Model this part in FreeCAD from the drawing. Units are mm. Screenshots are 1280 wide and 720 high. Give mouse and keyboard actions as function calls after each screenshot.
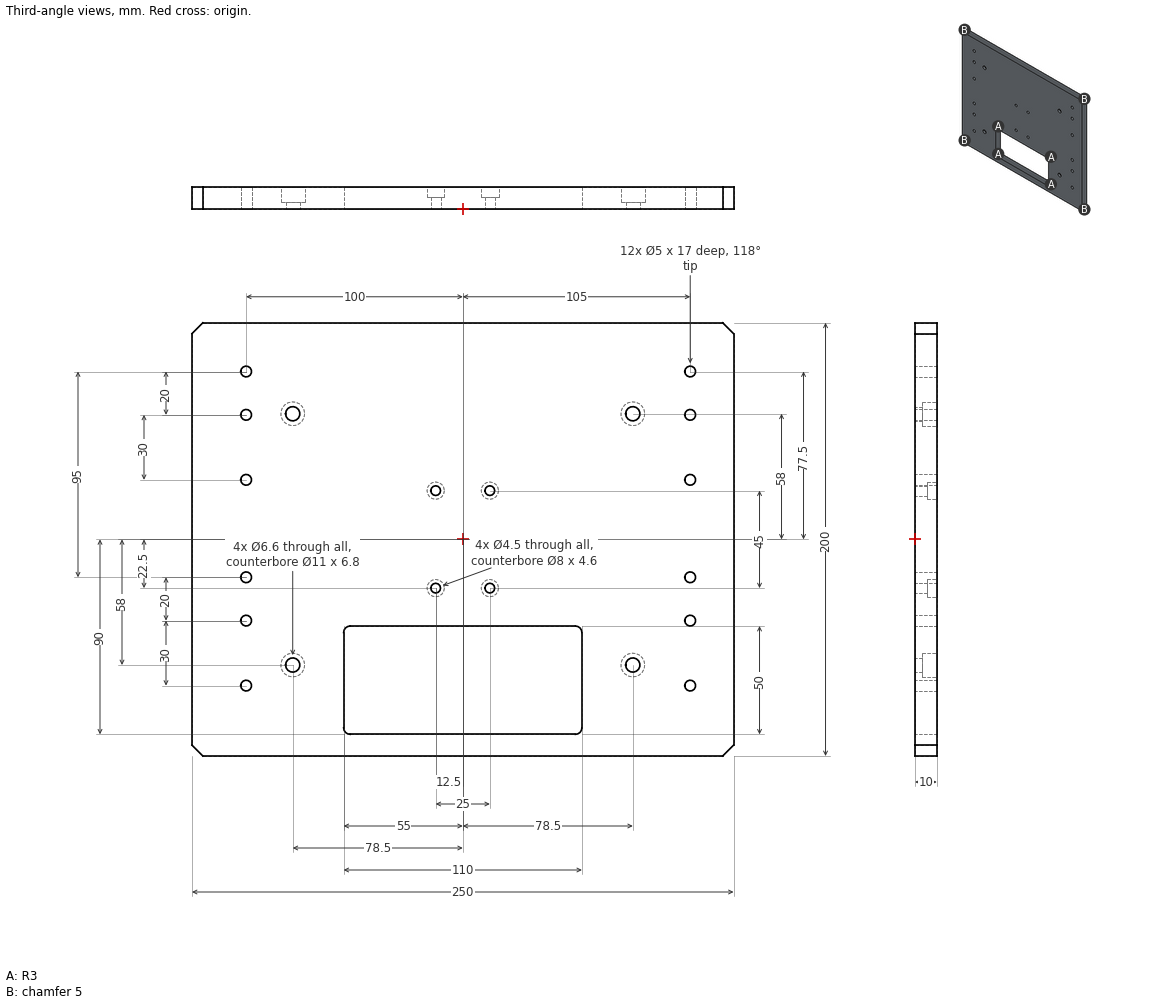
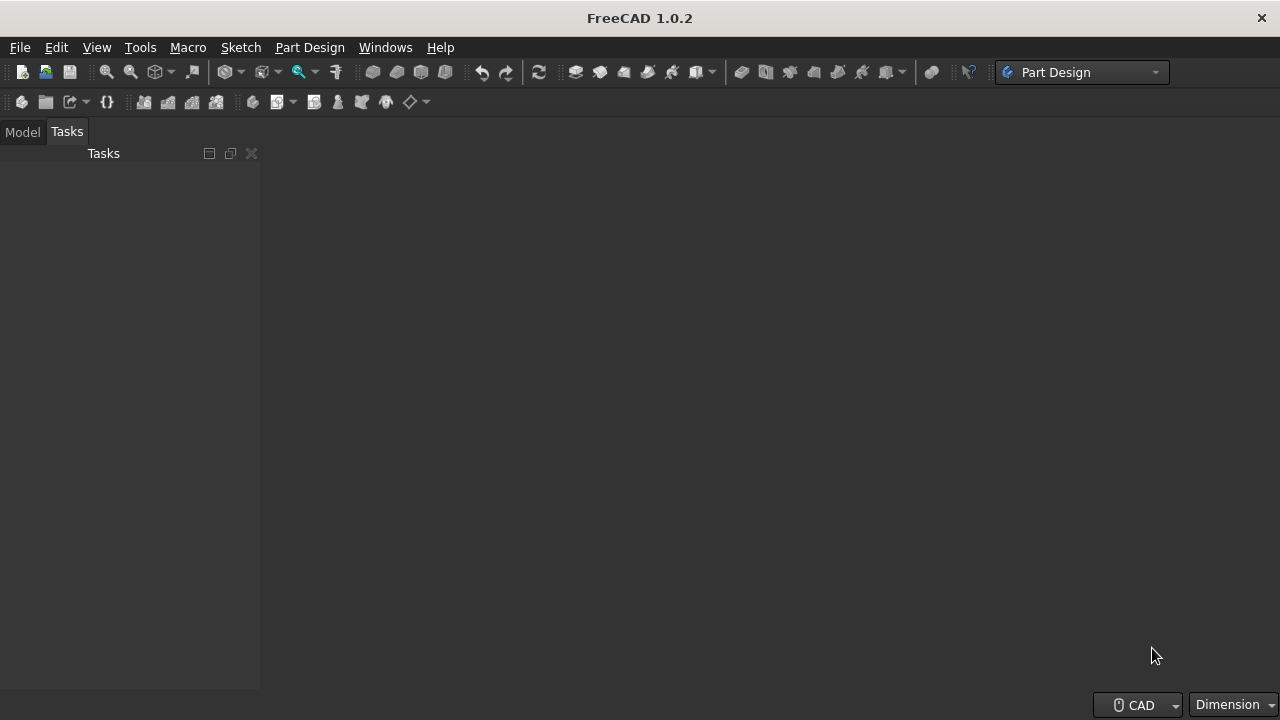
click(22, 72)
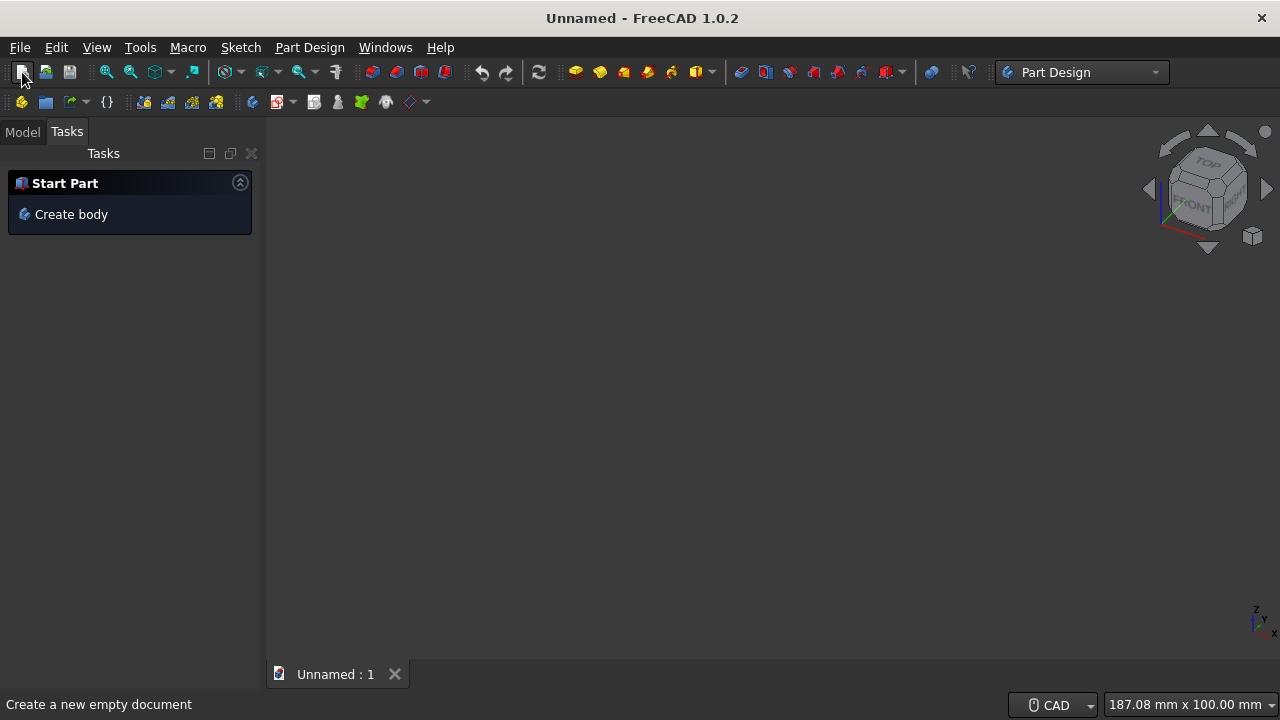
click(278, 102)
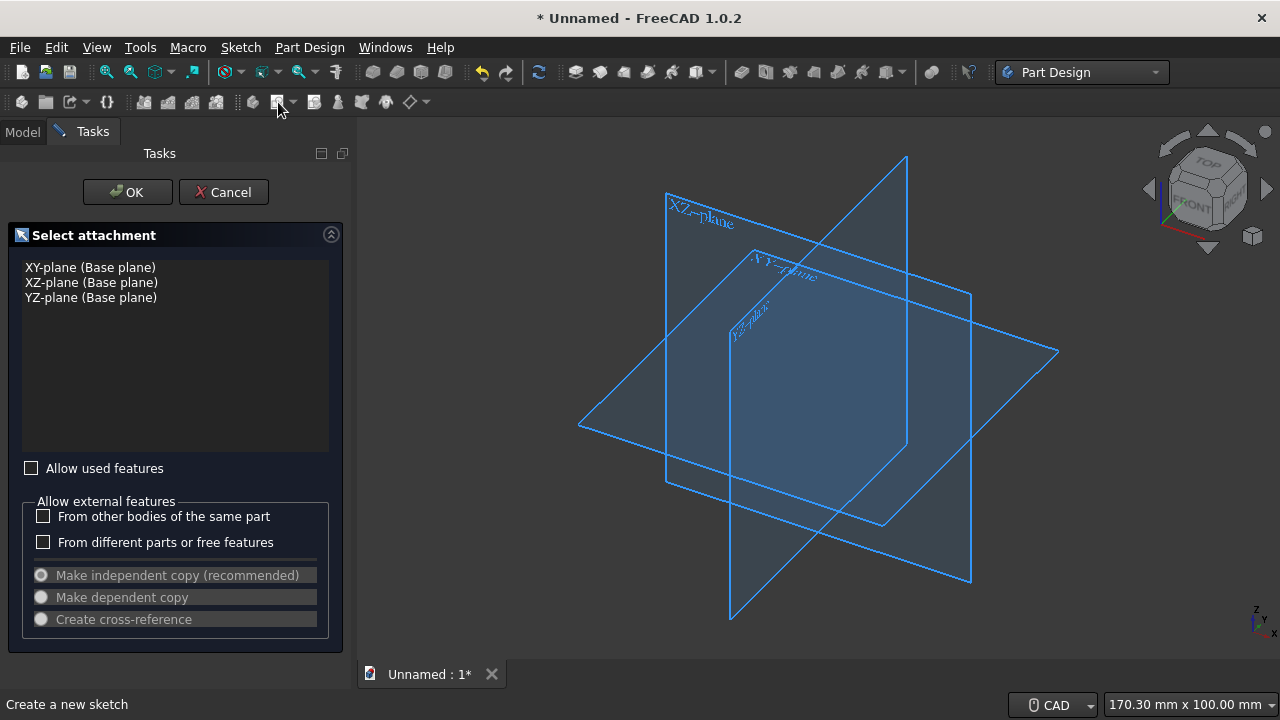
click(82, 282)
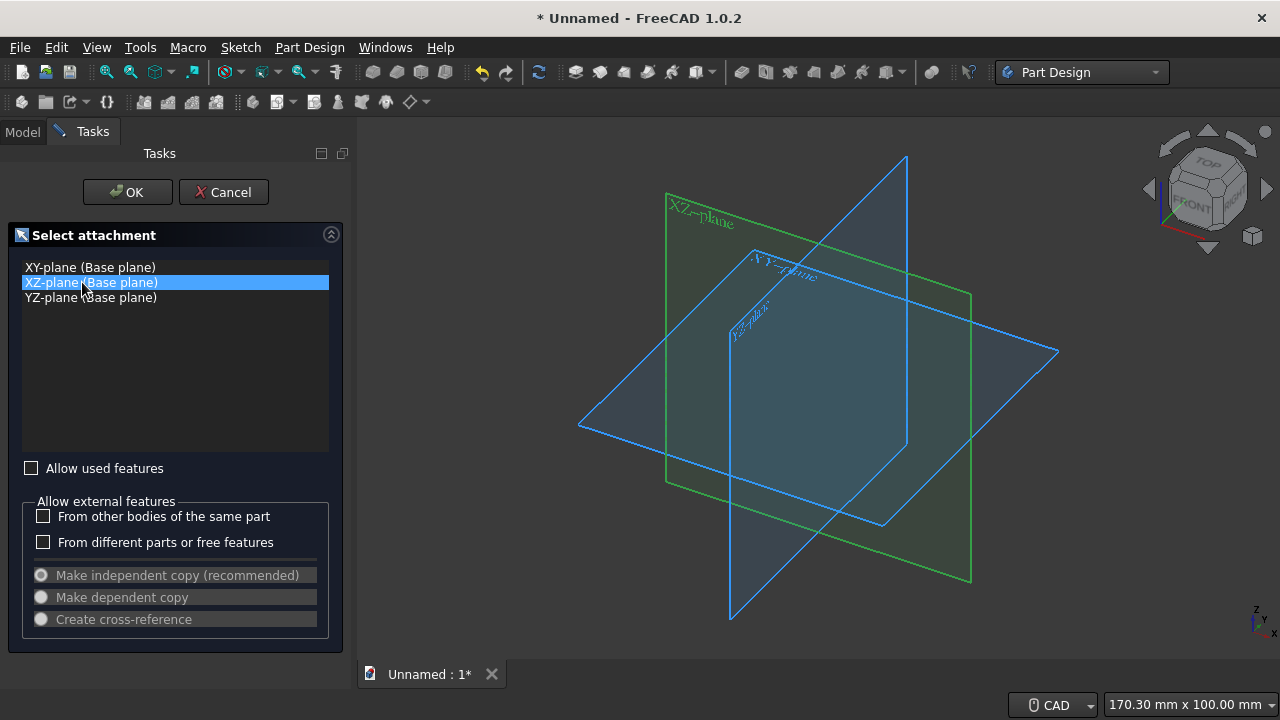
click(128, 192)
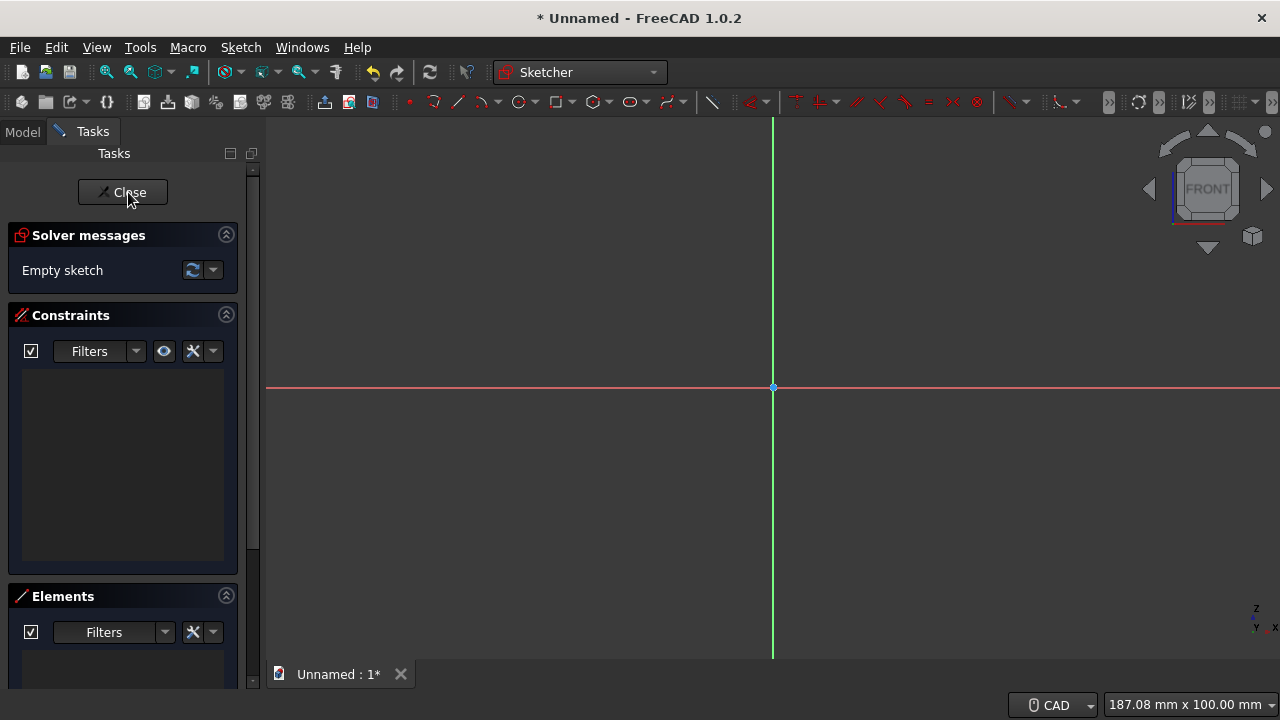
scroll(675, 388, down, 6)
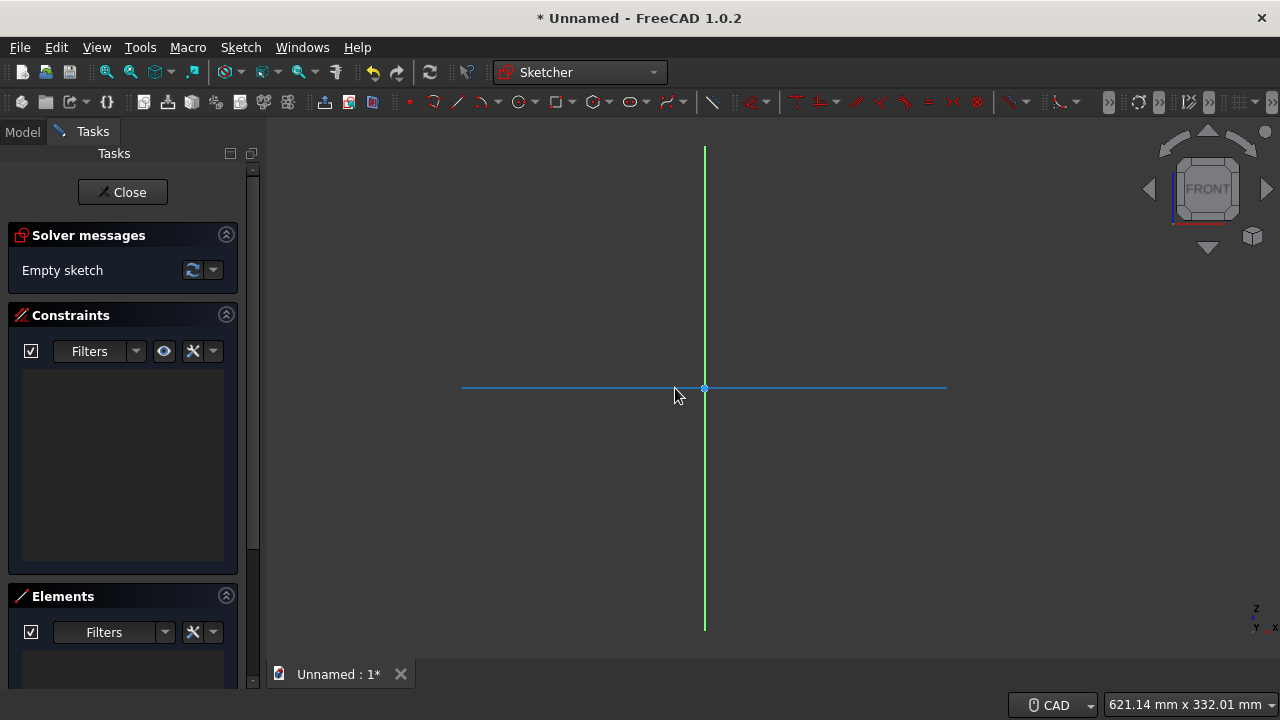
click(574, 102)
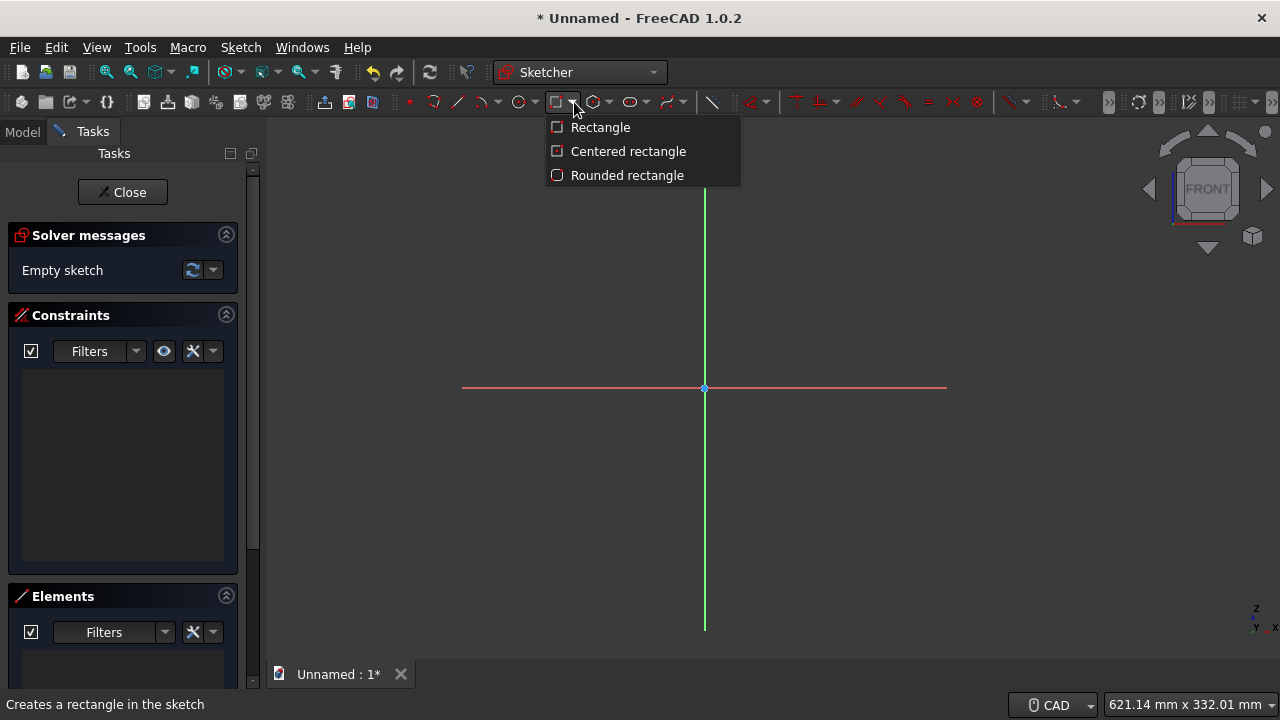
click(644, 151)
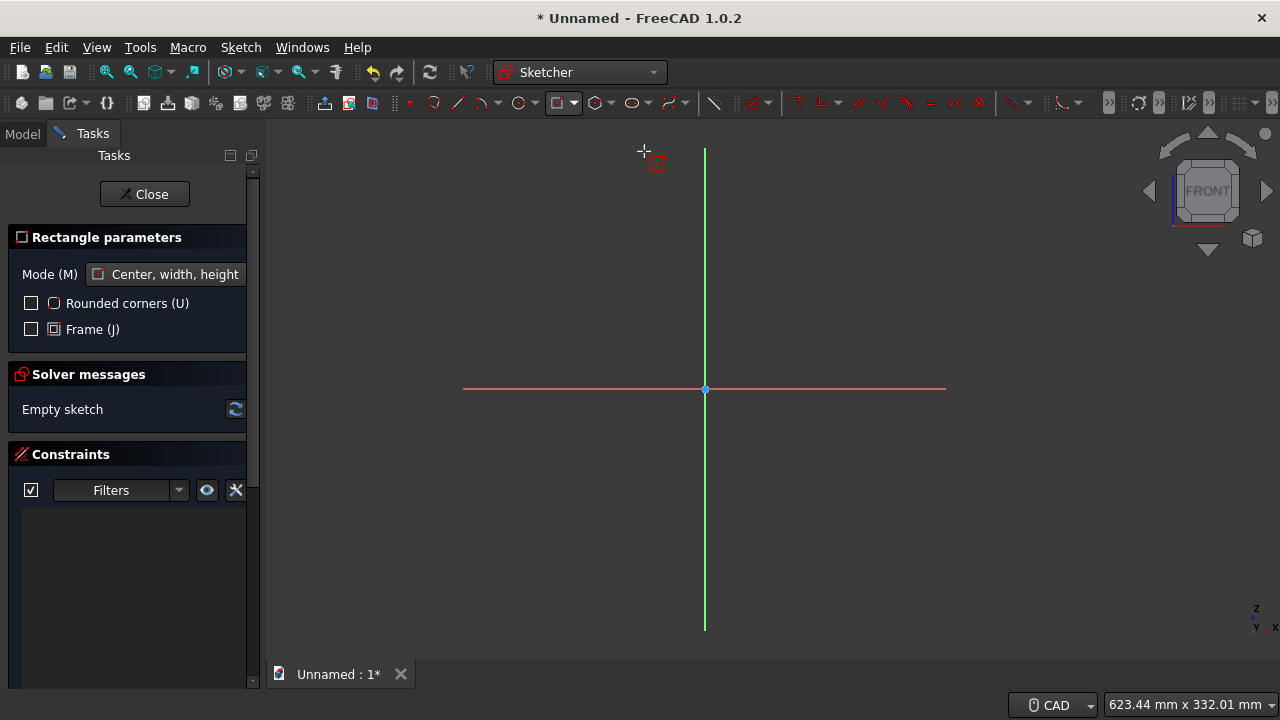
click(705, 389)
move(908, 227)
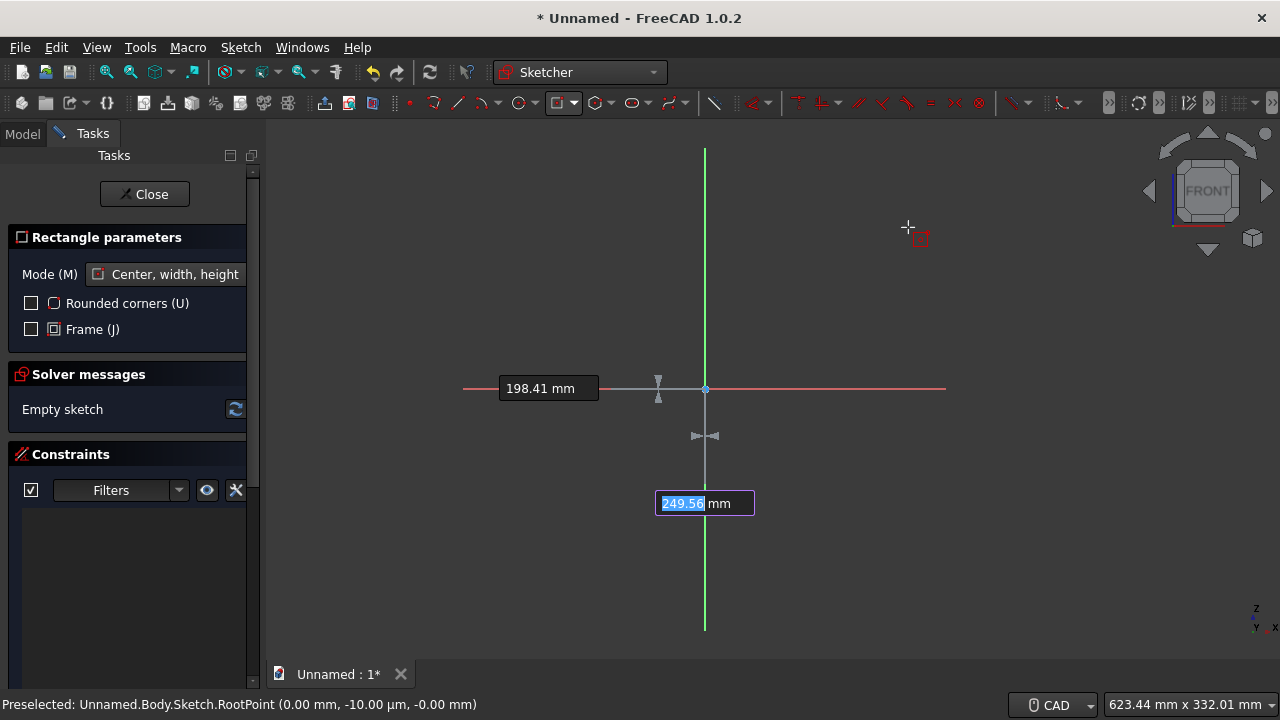
text(250)
key(Tab)
text(200)
key(Return)
key(Escape)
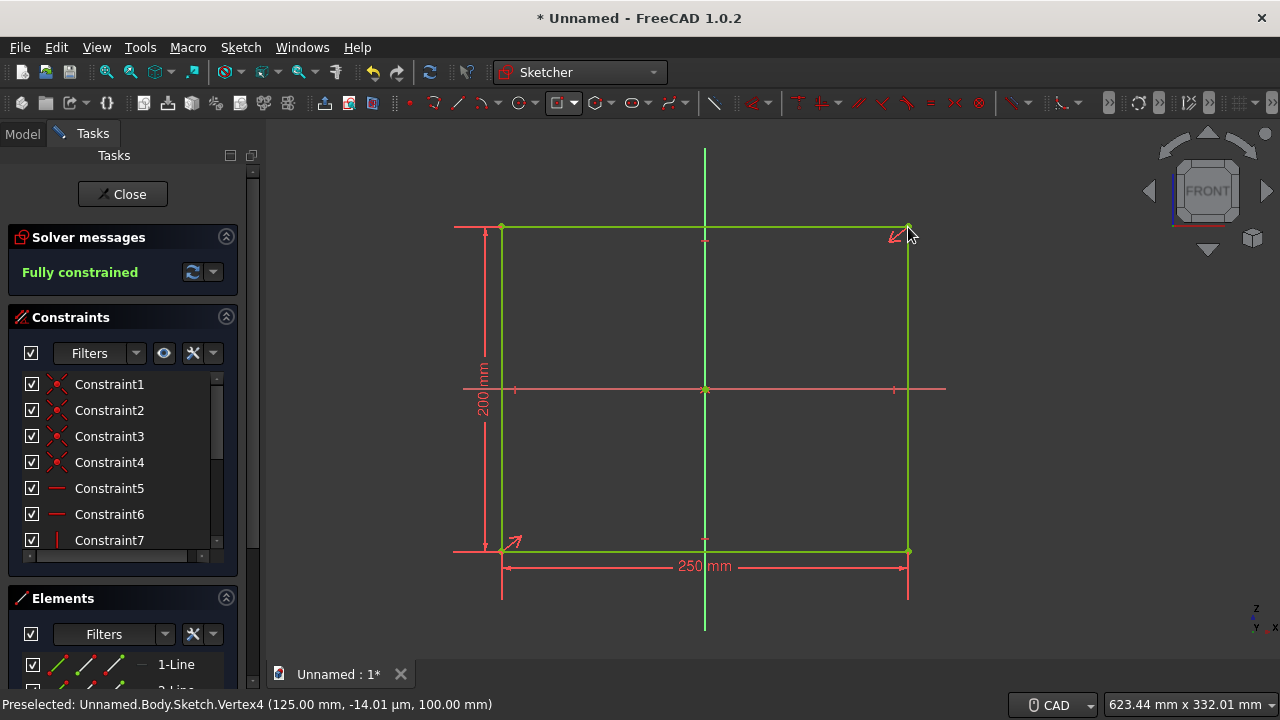
click(123, 194)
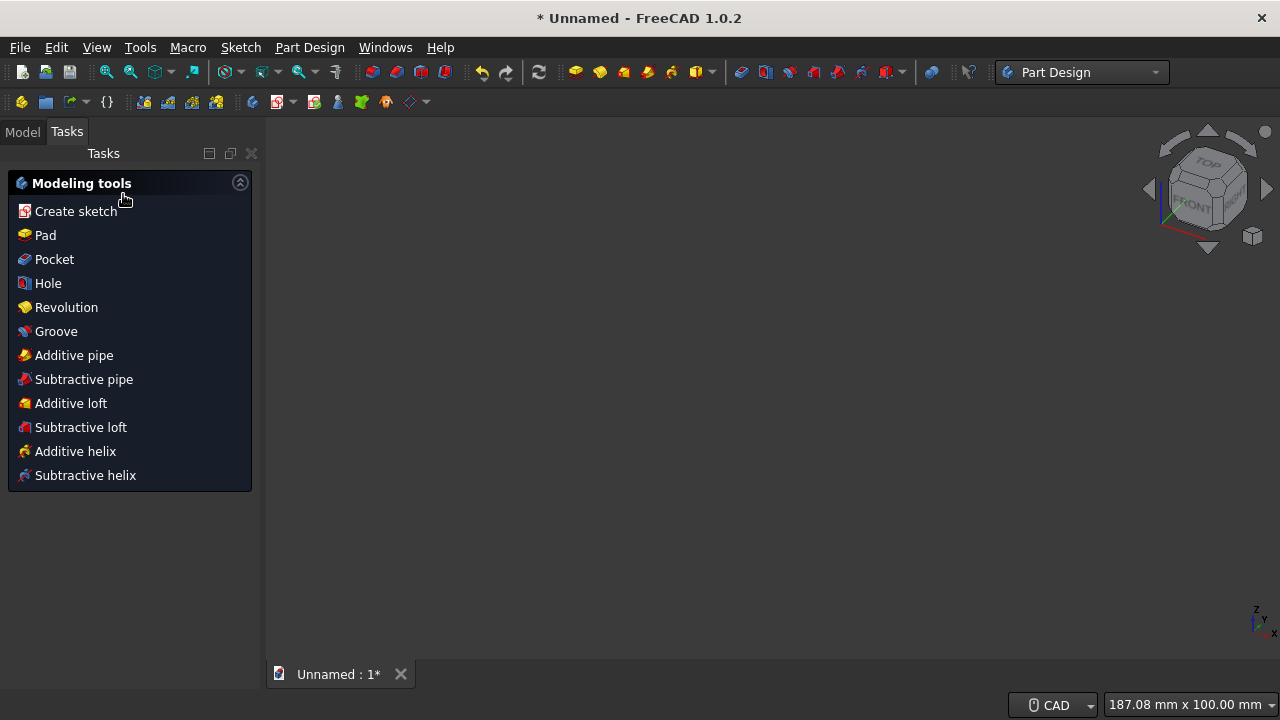
click(576, 72)